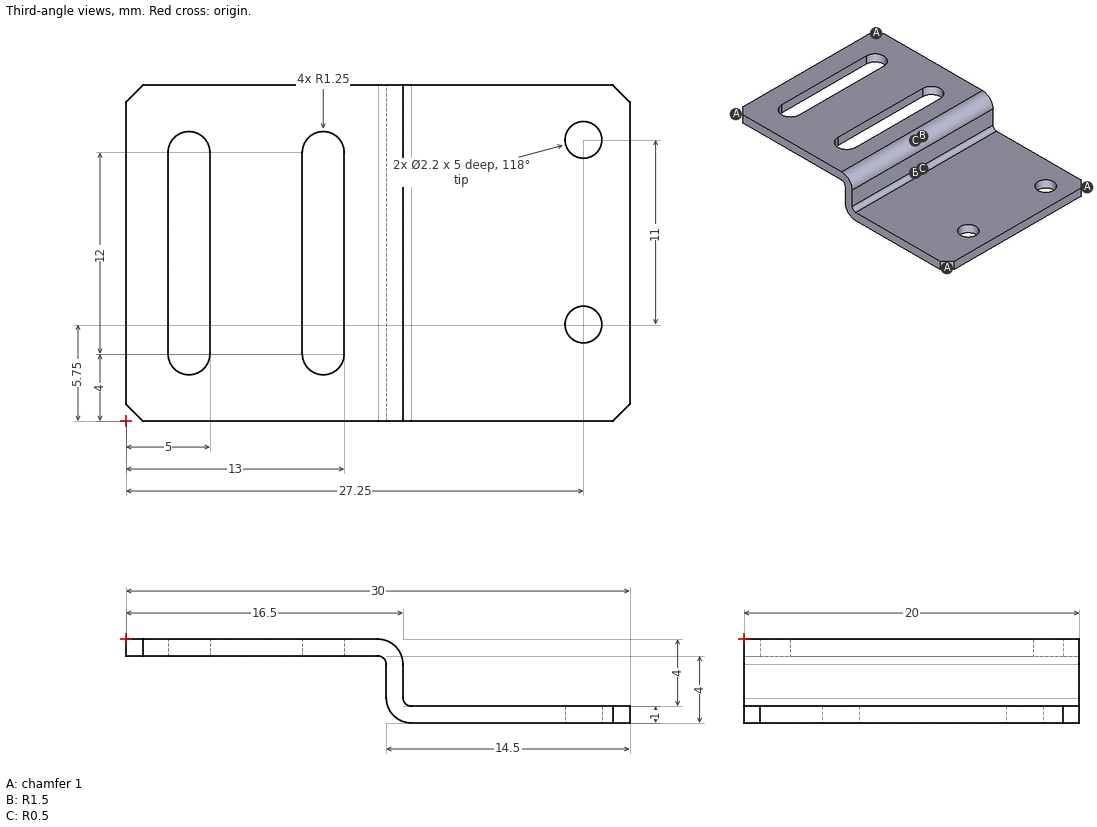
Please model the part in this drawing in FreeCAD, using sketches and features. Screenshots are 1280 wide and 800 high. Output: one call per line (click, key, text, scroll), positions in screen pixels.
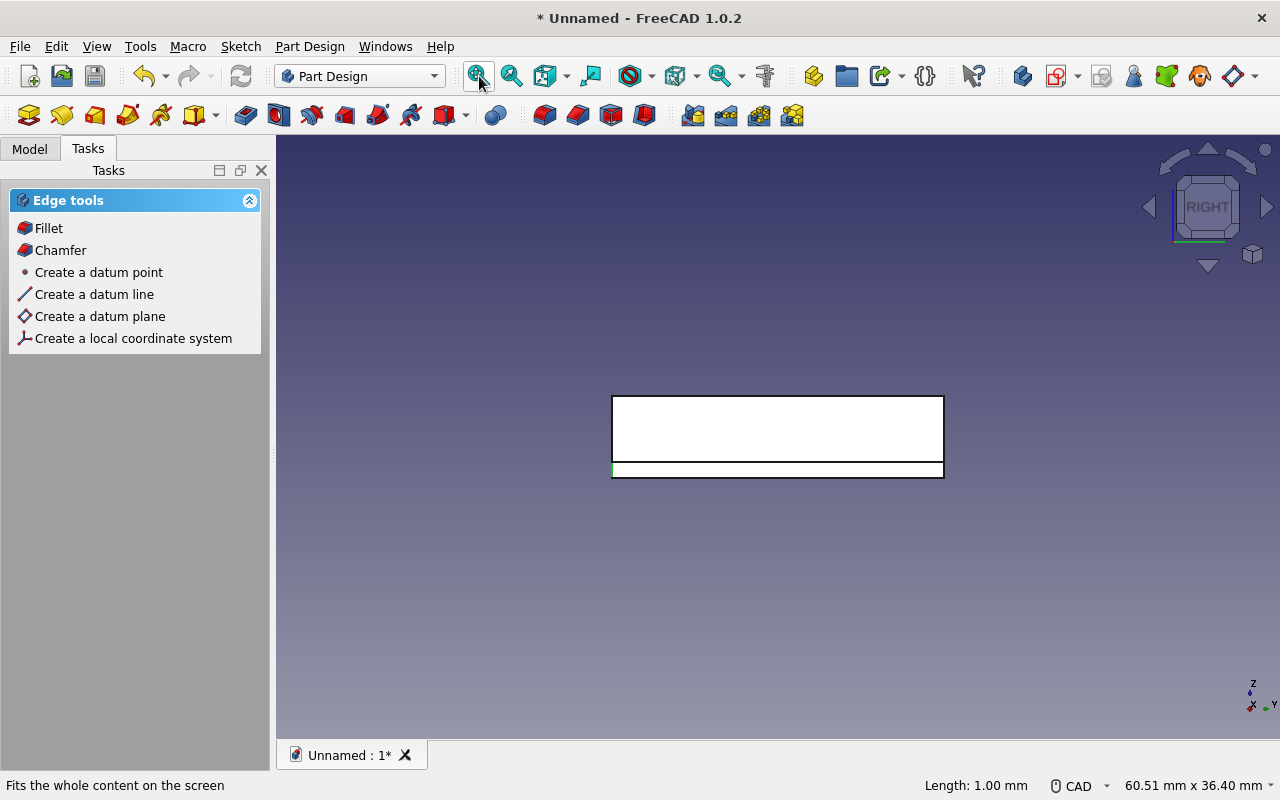
click(479, 76)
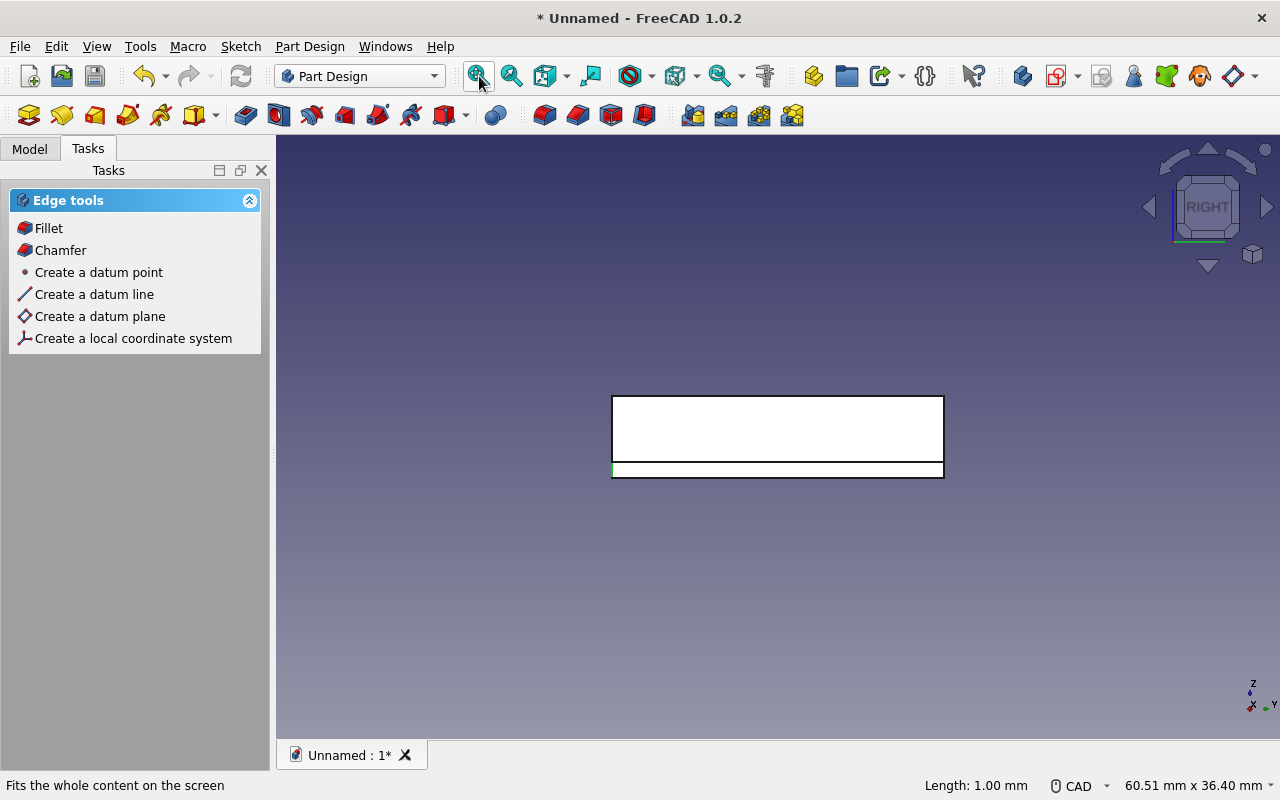
click(944, 469, ctrl)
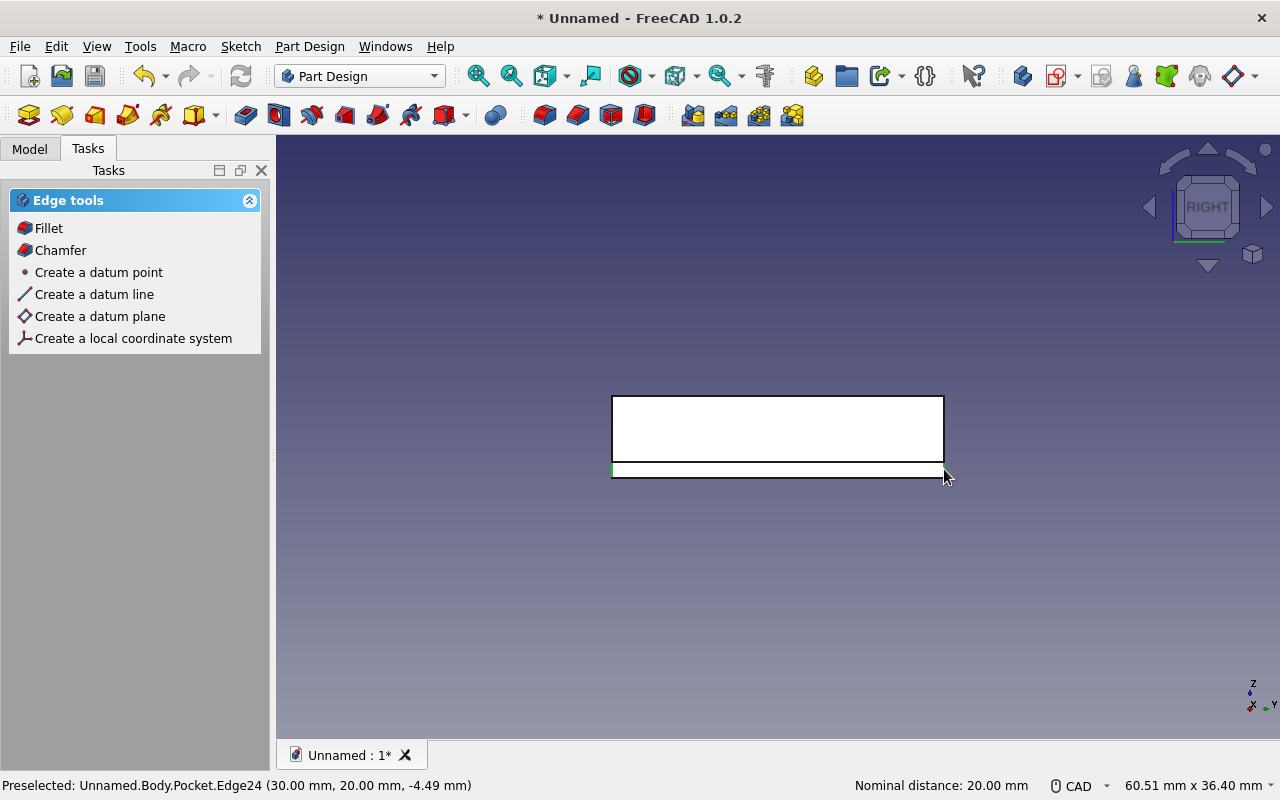
scroll(612, 403, up, 5)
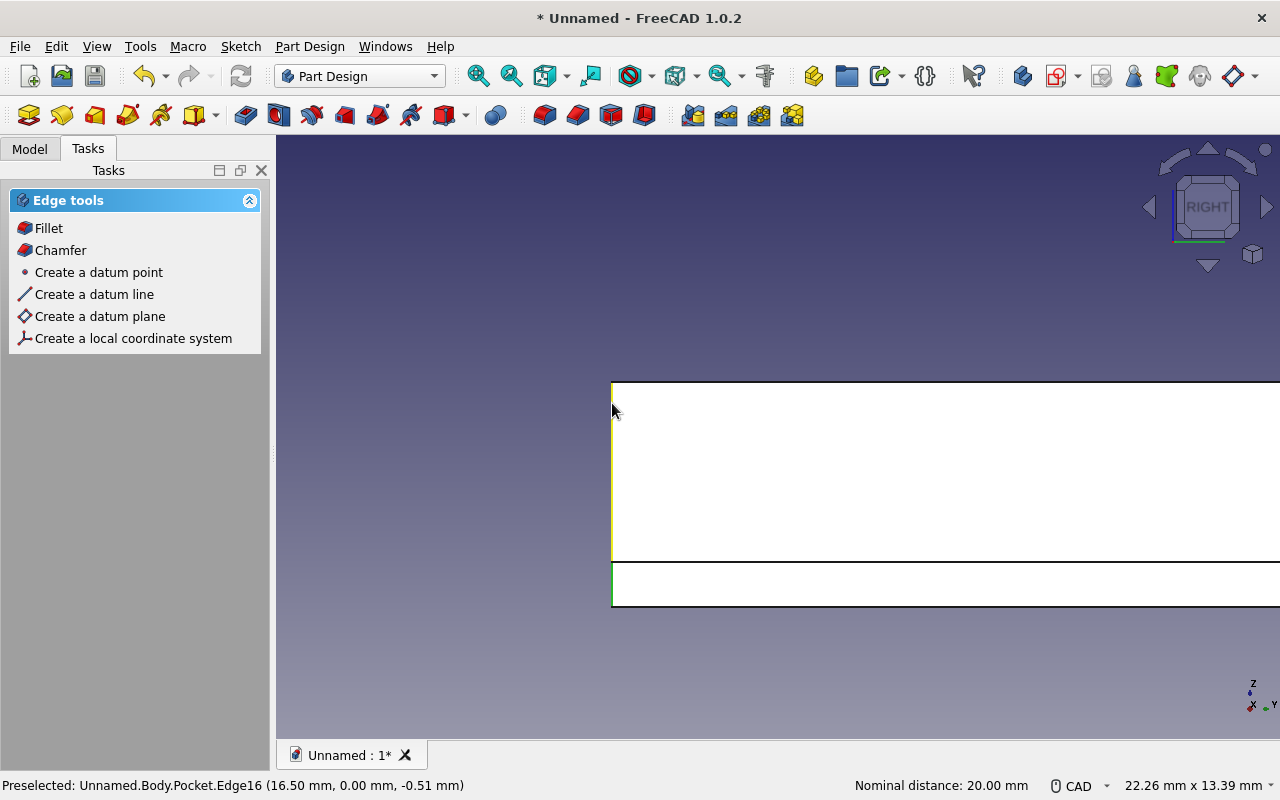
click(479, 76)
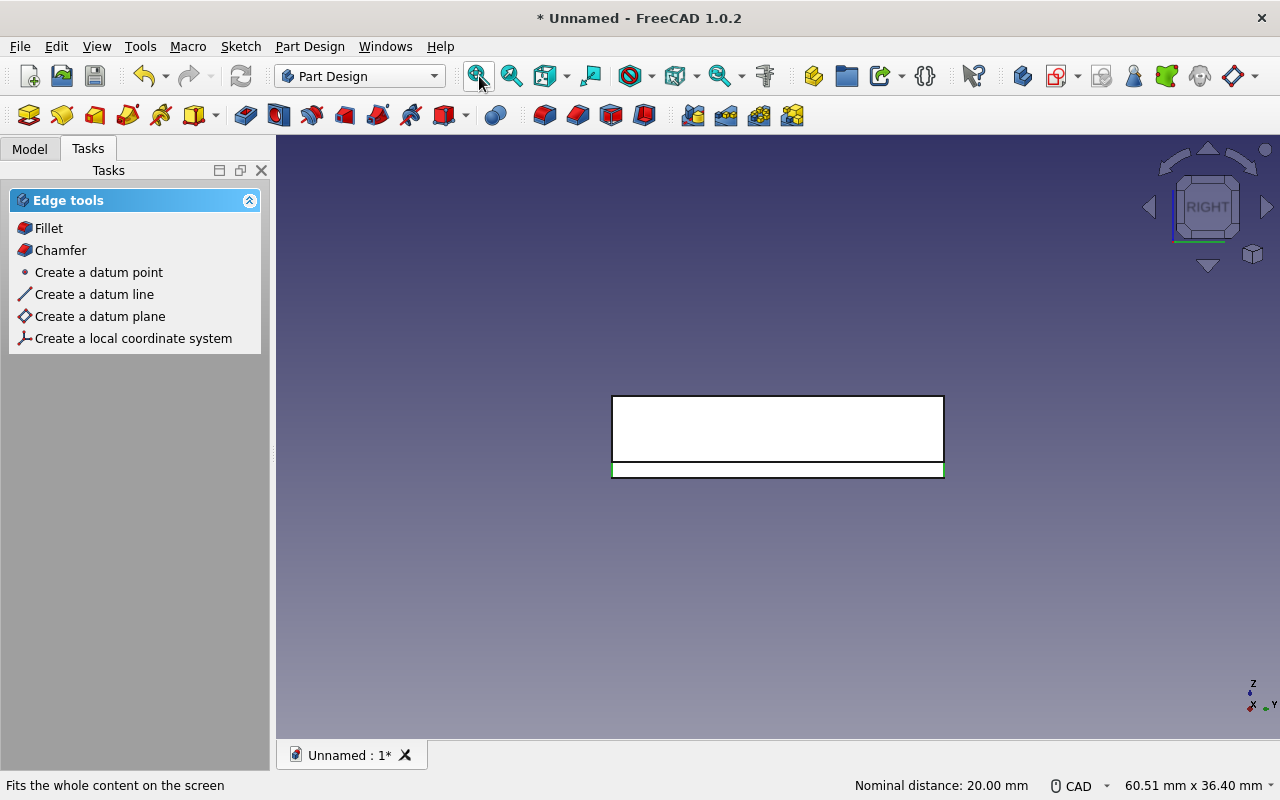
key(5)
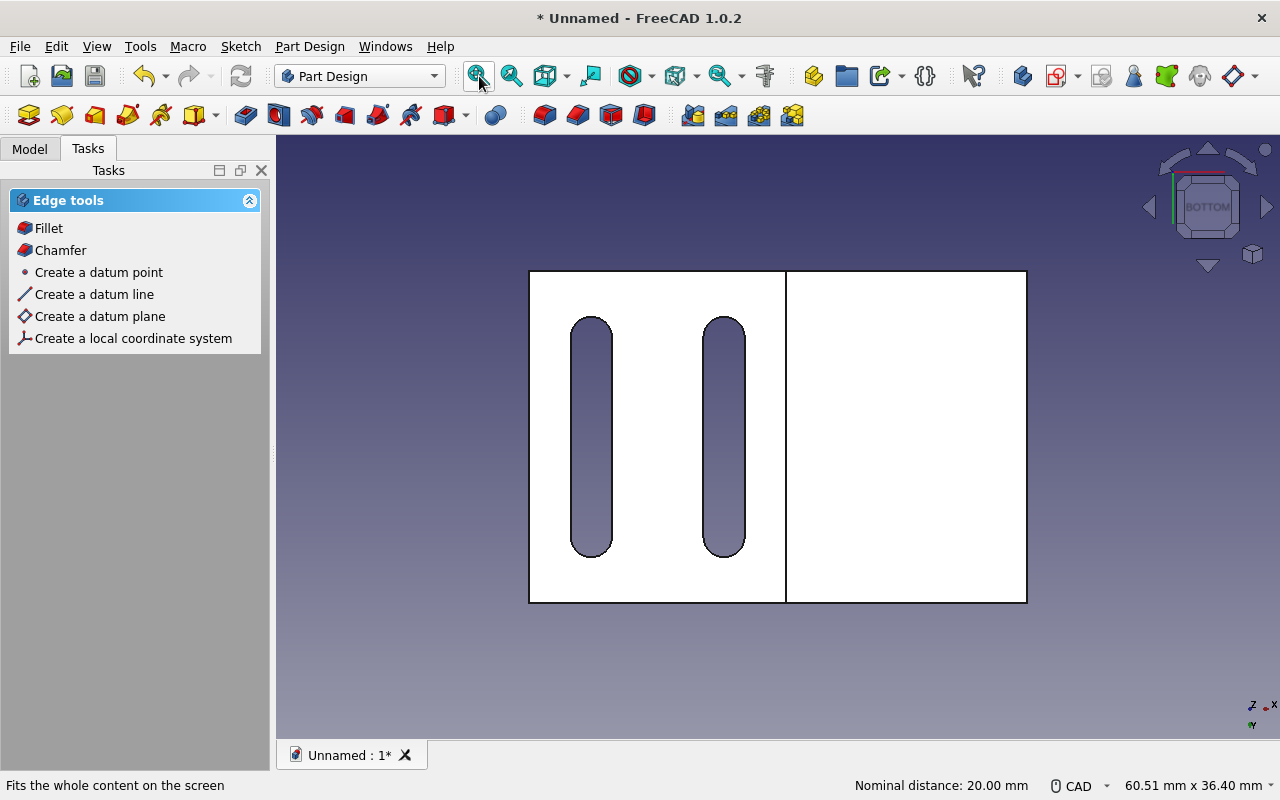
scroll(529, 270, up, 5)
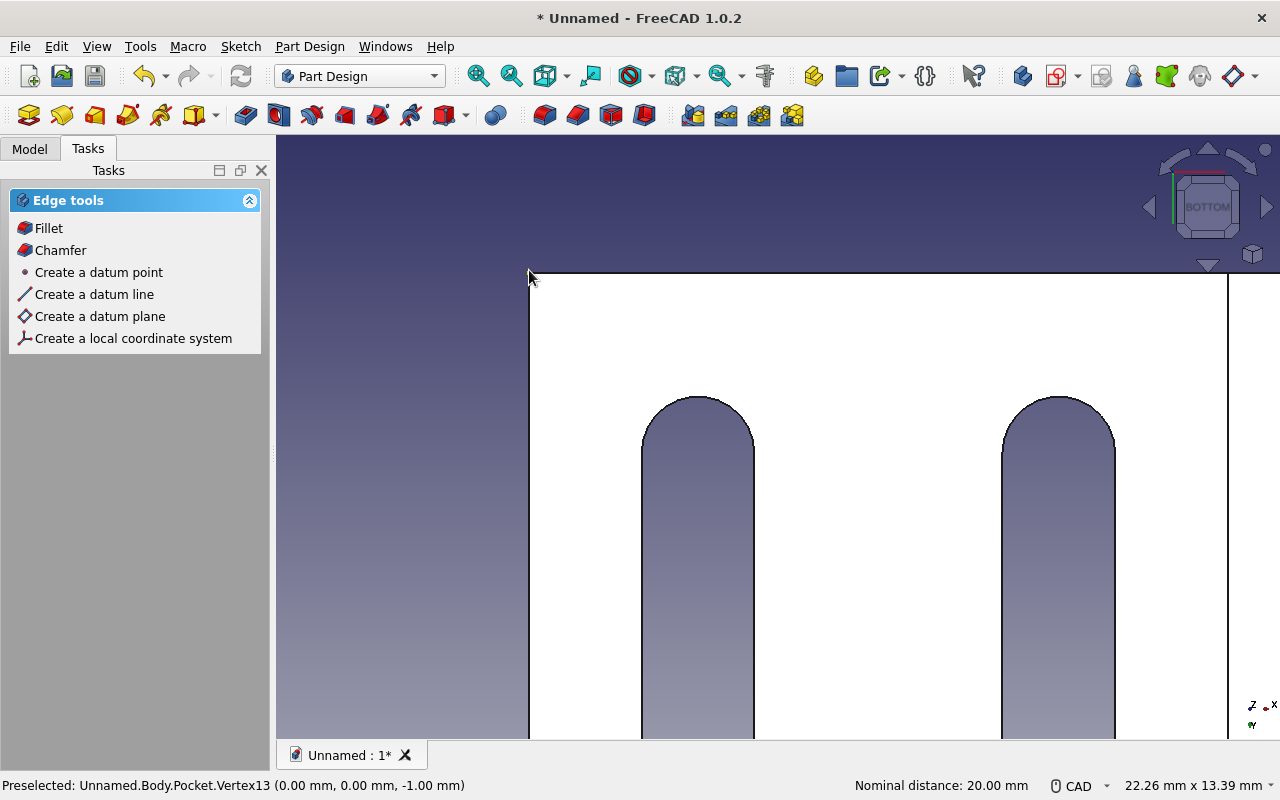
click(479, 76)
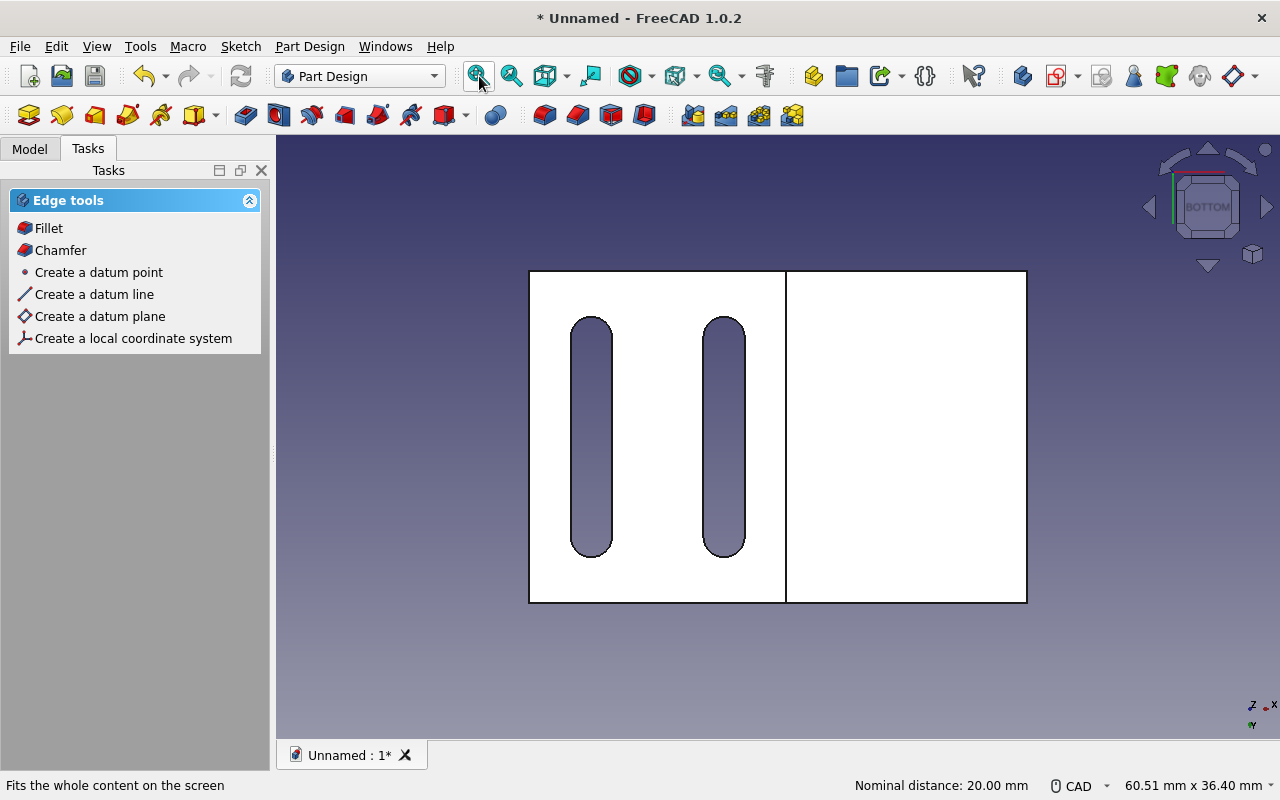
key(4)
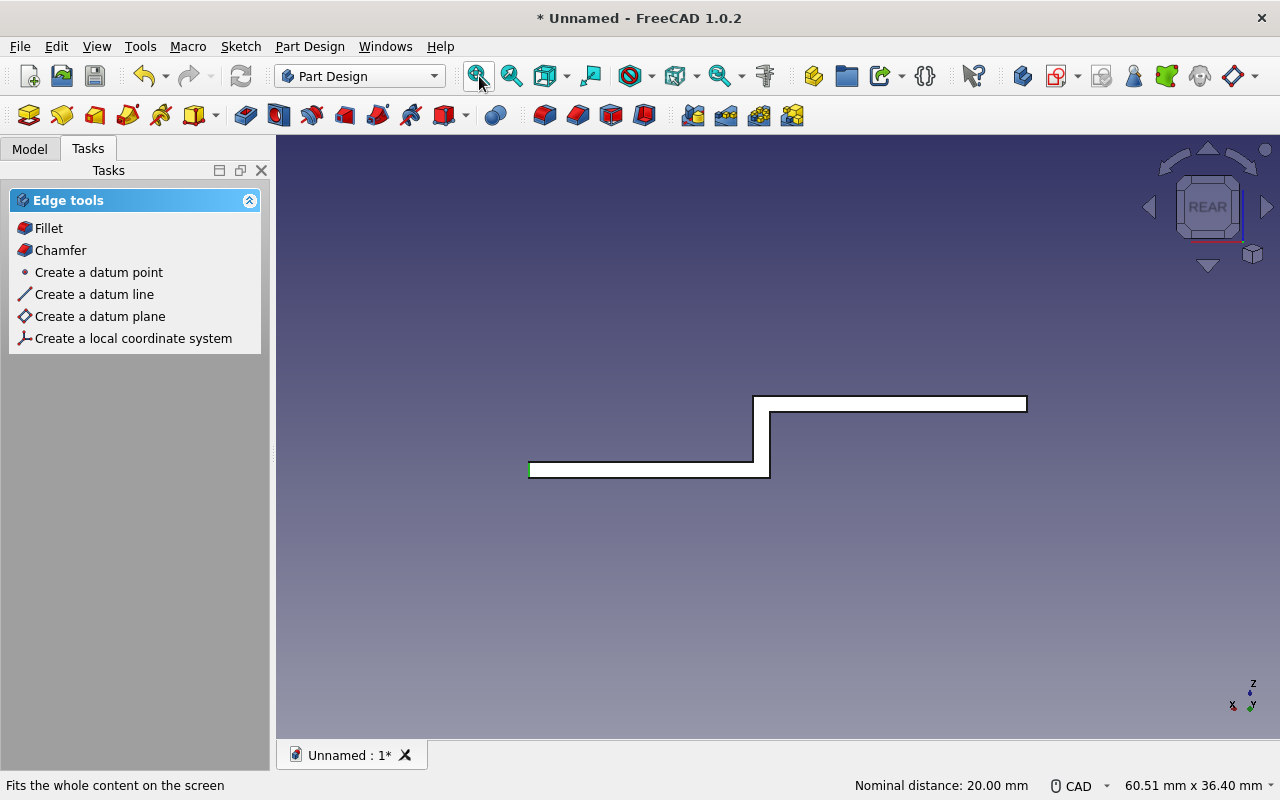
click(1027, 403, ctrl)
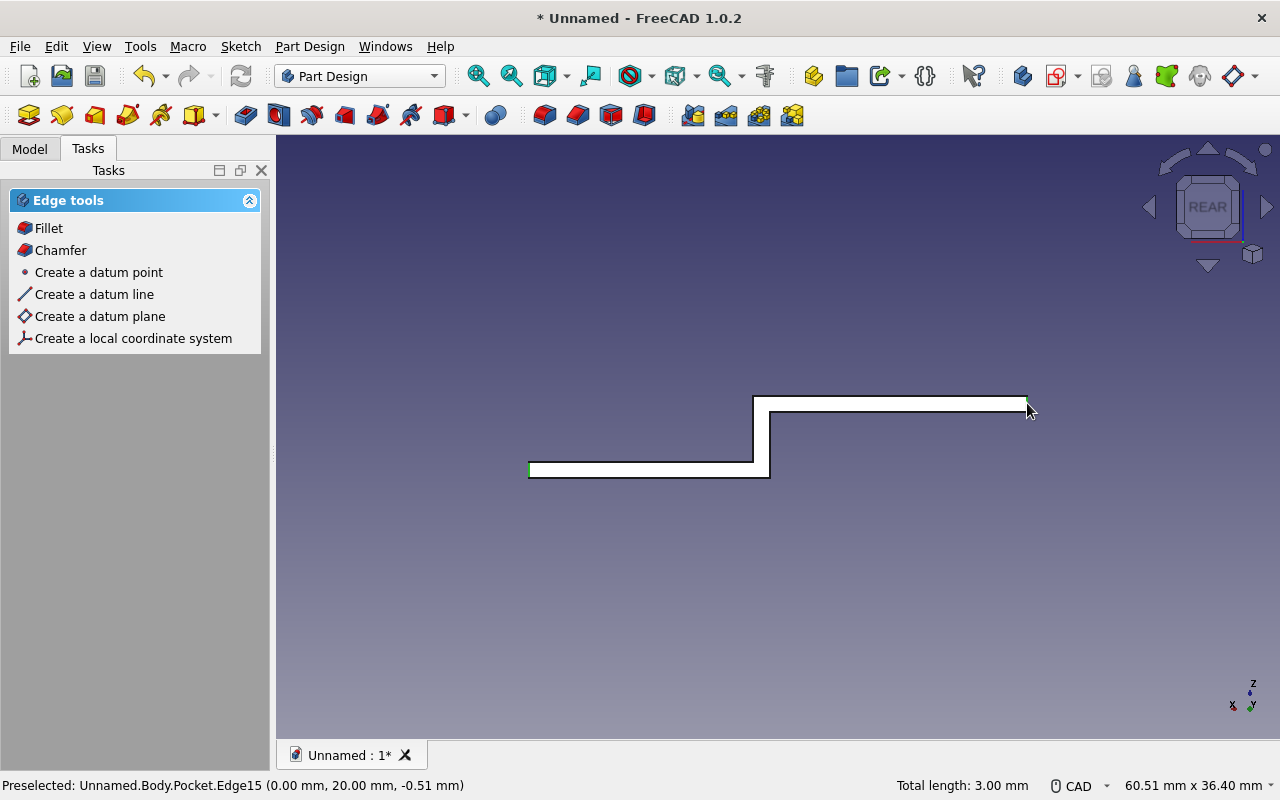
scroll(1027, 403, up, 5)